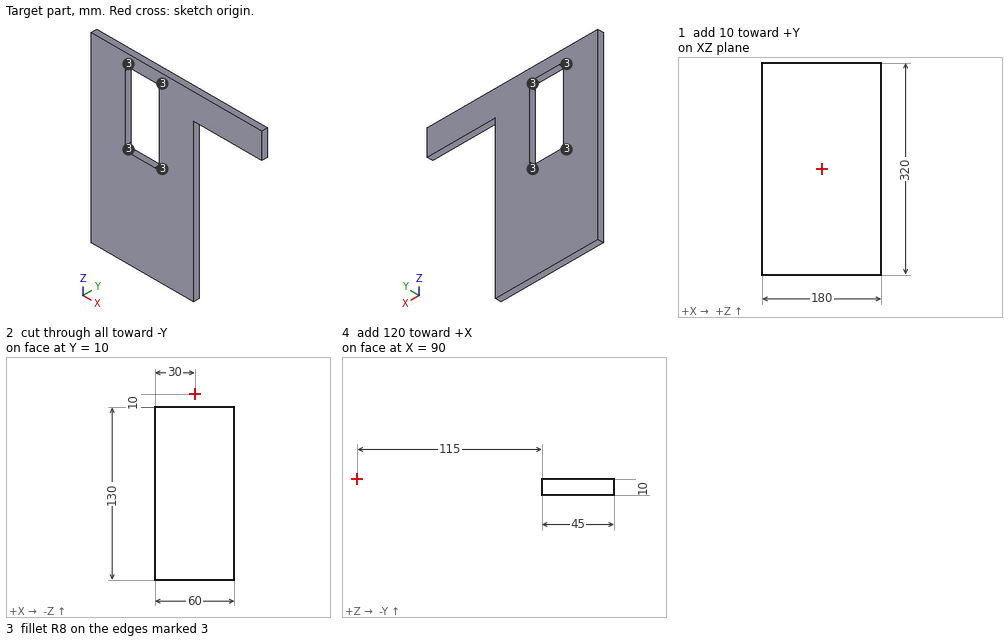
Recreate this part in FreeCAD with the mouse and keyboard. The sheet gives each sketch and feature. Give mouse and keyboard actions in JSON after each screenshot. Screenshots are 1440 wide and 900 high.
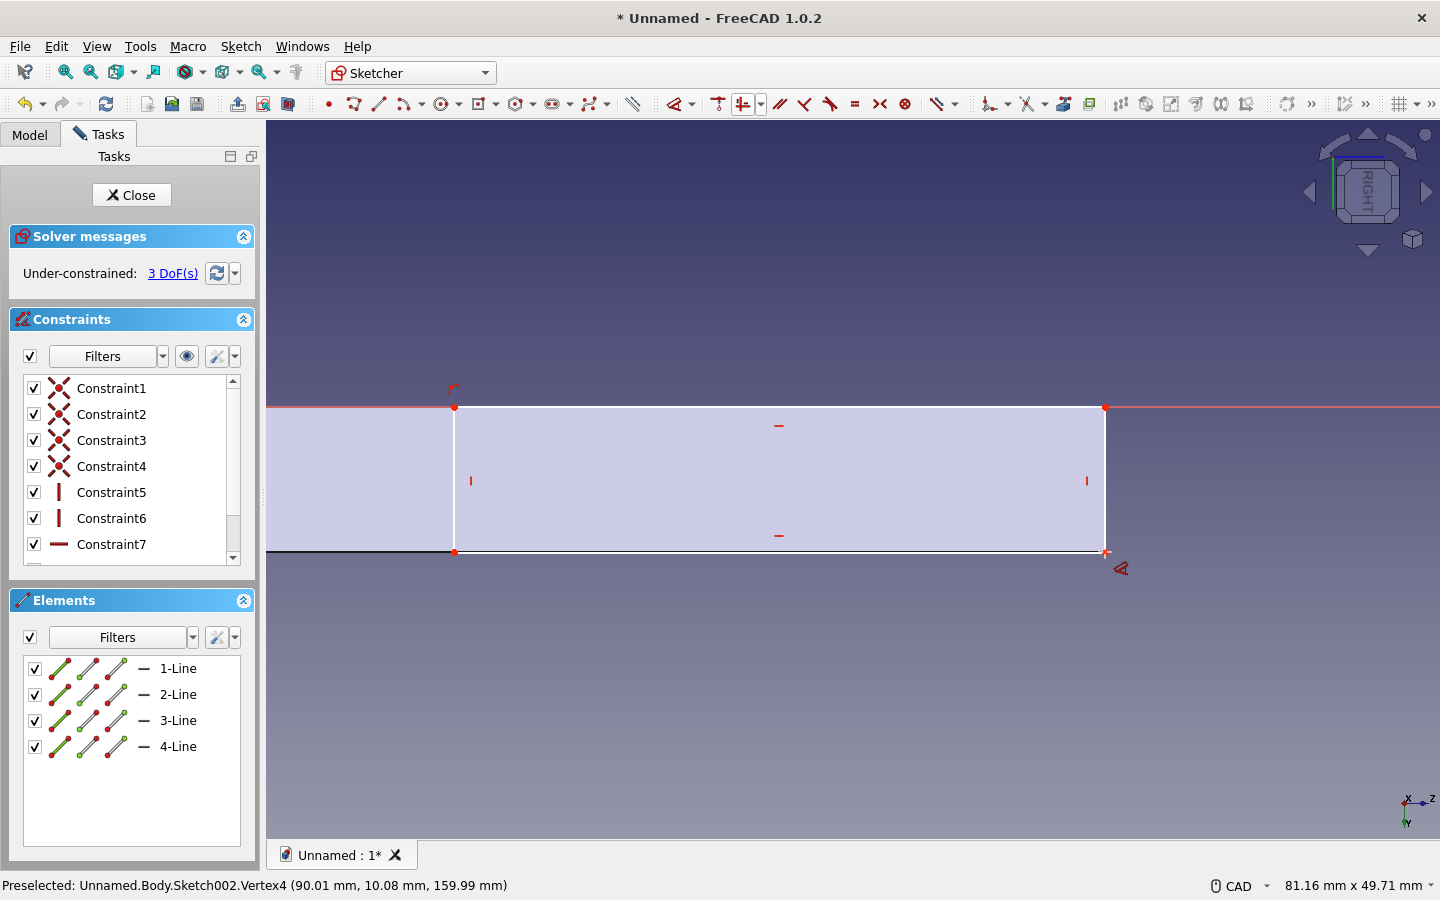
{"action": "left_click", "coordinate": [454, 451]}
{"action": "left_click", "coordinate": [420, 480]}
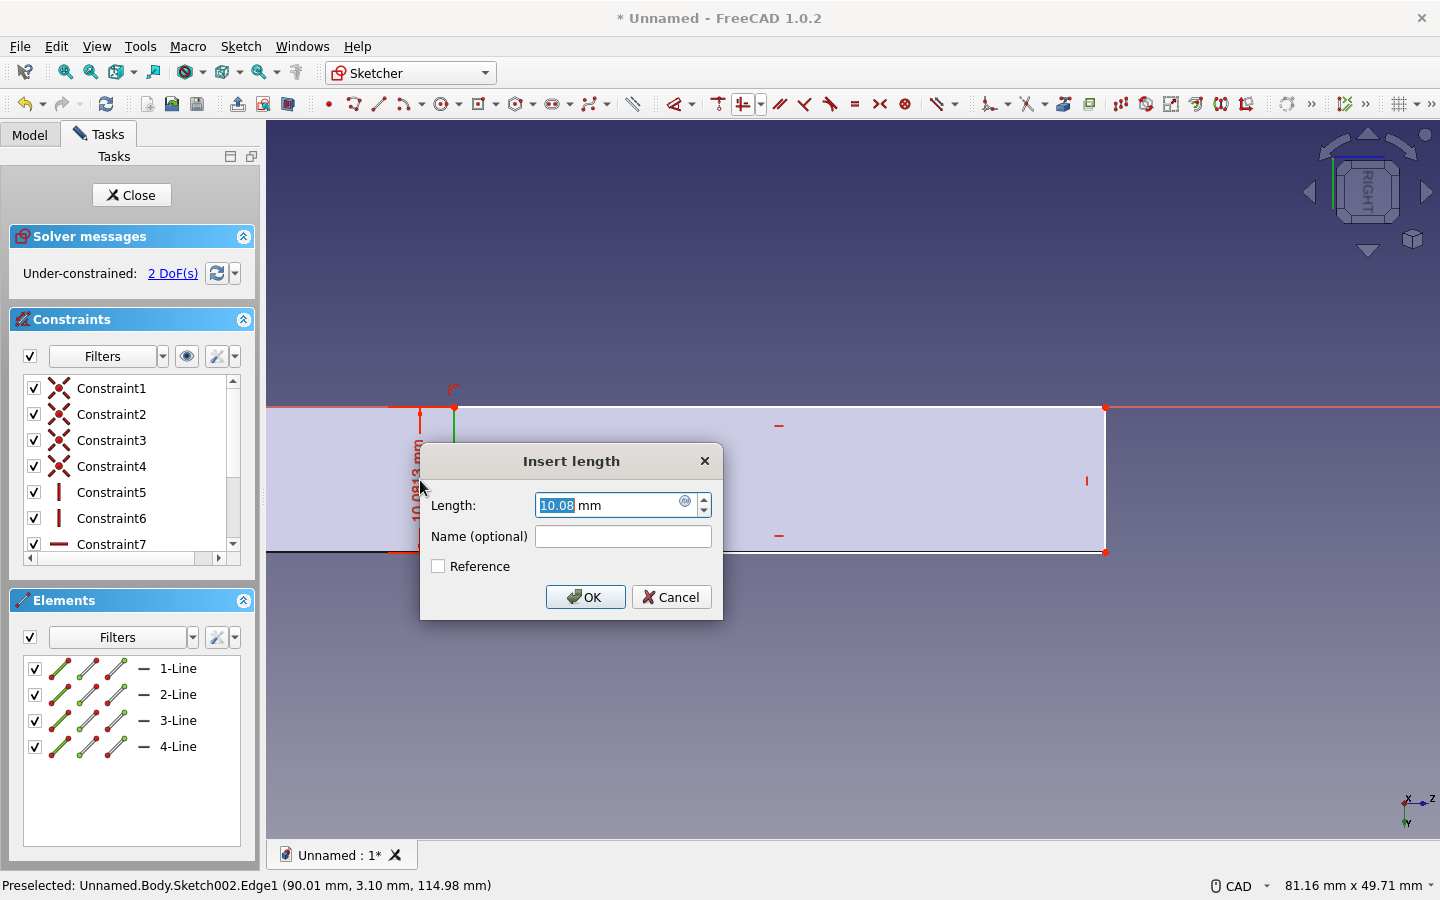
{"action": "type", "text": "10"}
{"action": "key", "text": "Return"}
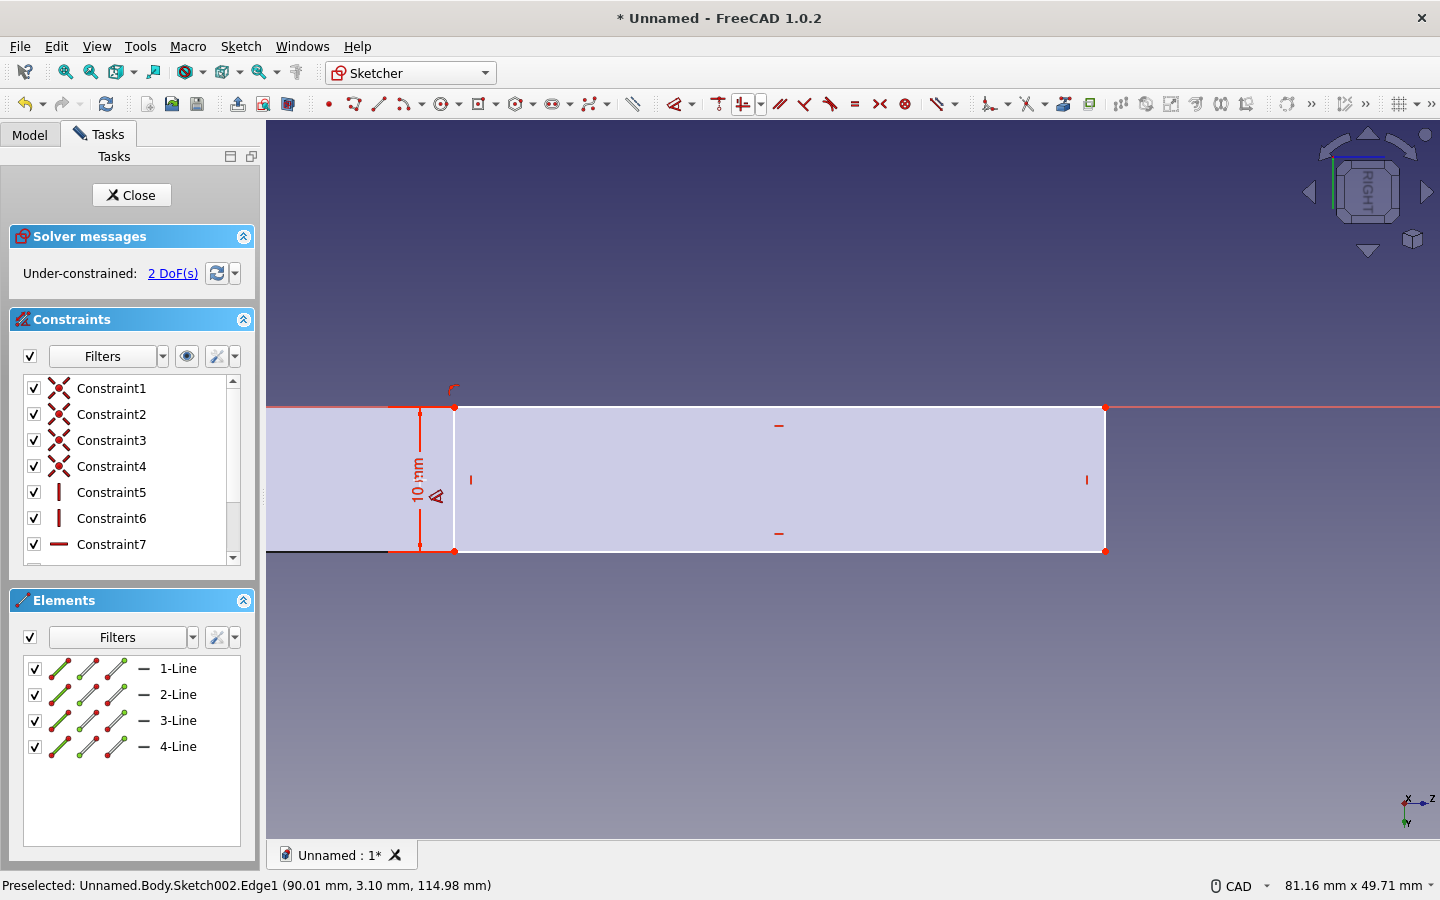
{"action": "left_click", "coordinate": [649, 552]}
{"action": "left_click", "coordinate": [779, 586]}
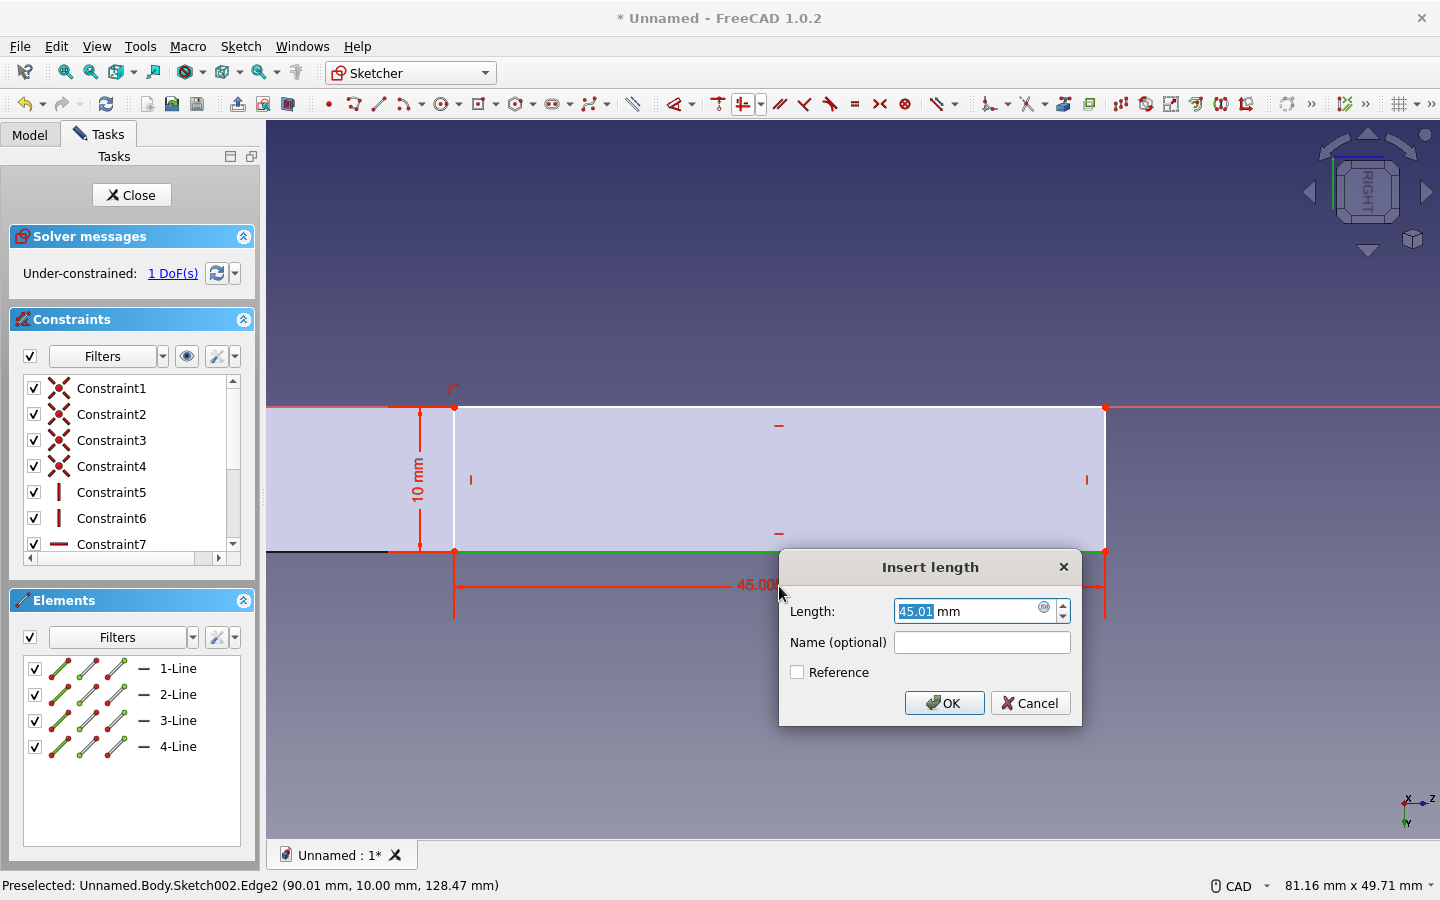
{"action": "type", "text": "45"}
{"action": "key", "text": "Return"}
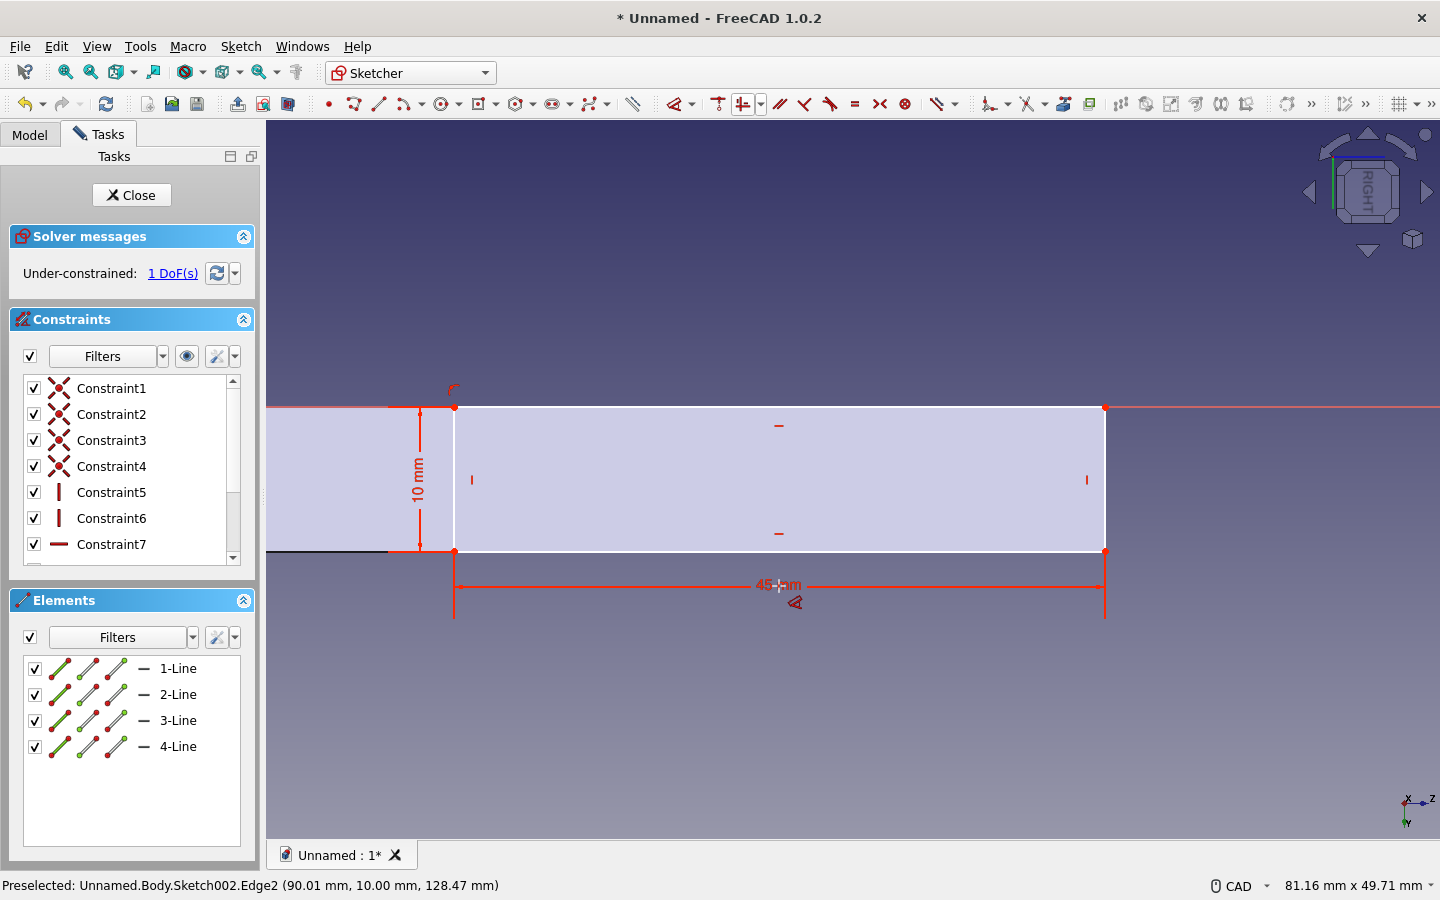
{"action": "left_click", "coordinate": [454, 407]}
{"action": "left_click", "coordinate": [374, 373]}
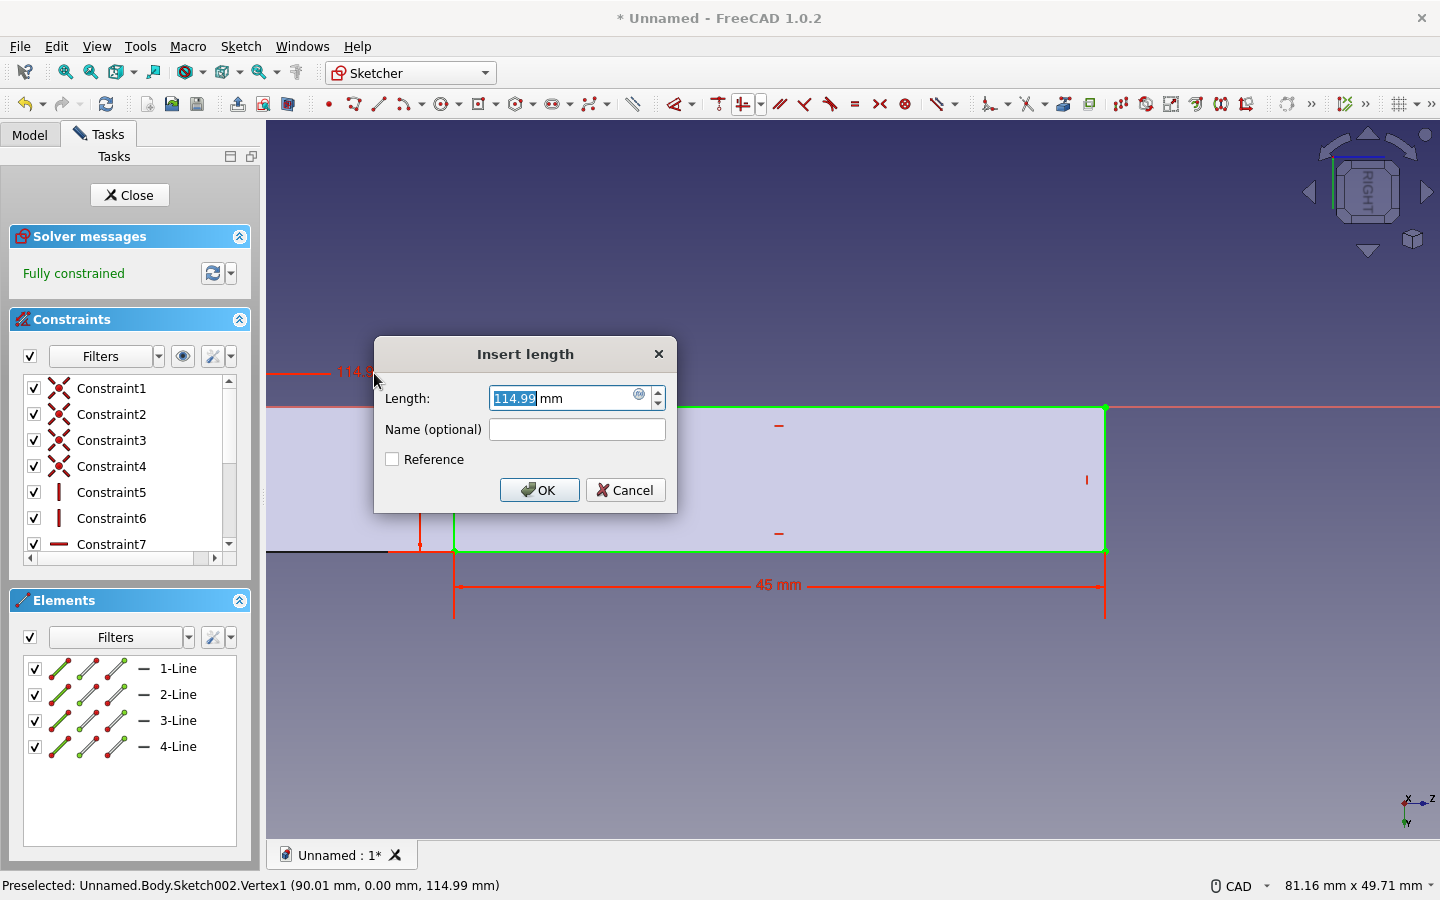
{"action": "type", "text": "115"}
{"action": "key", "text": "Return"}
{"action": "key", "text": "Escape"}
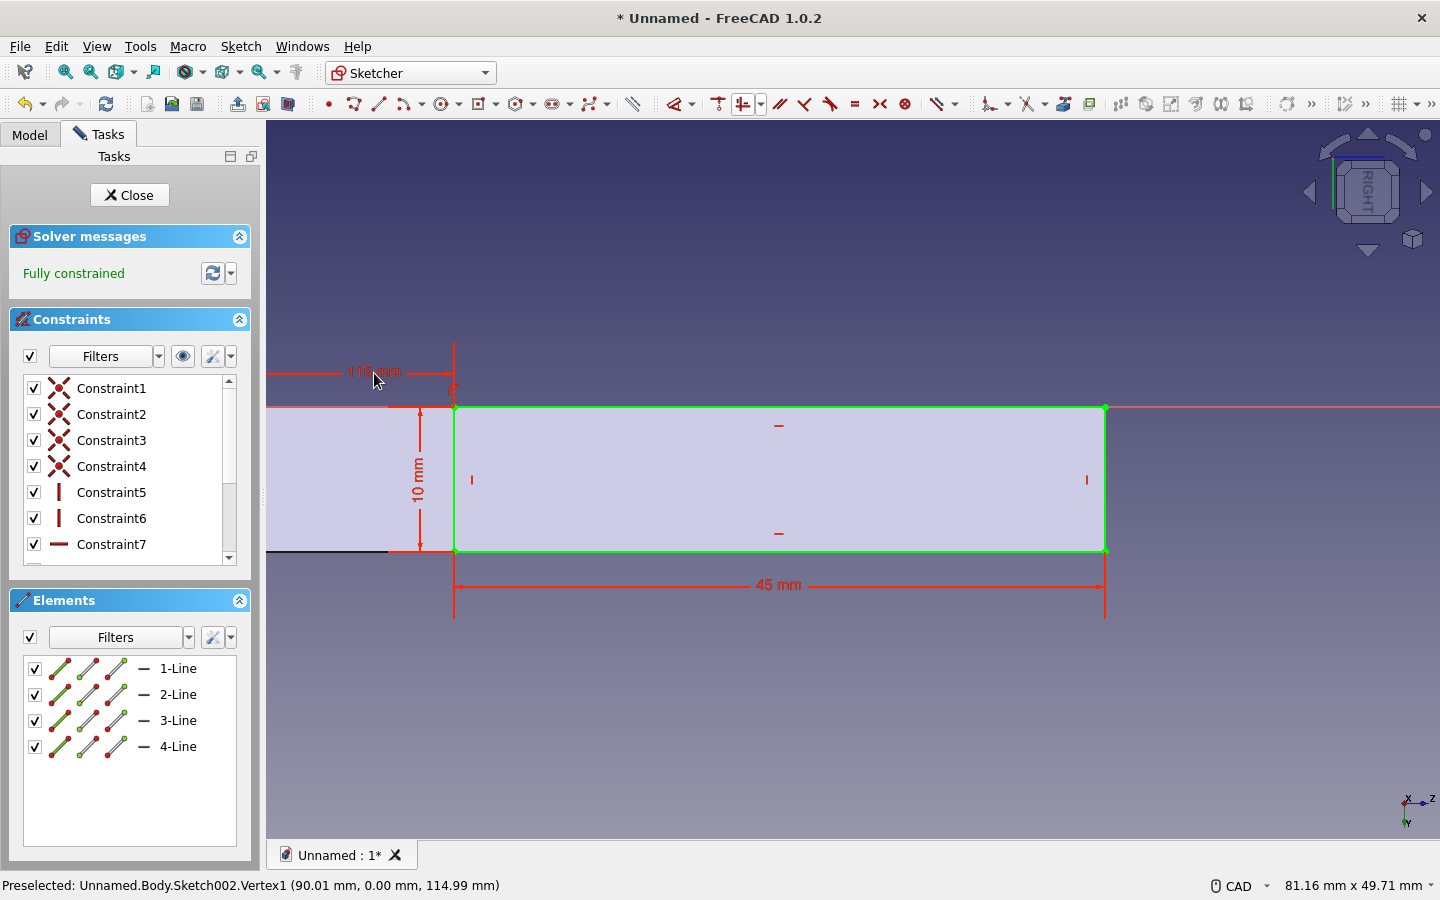
{"action": "left_click", "coordinate": [130, 195]}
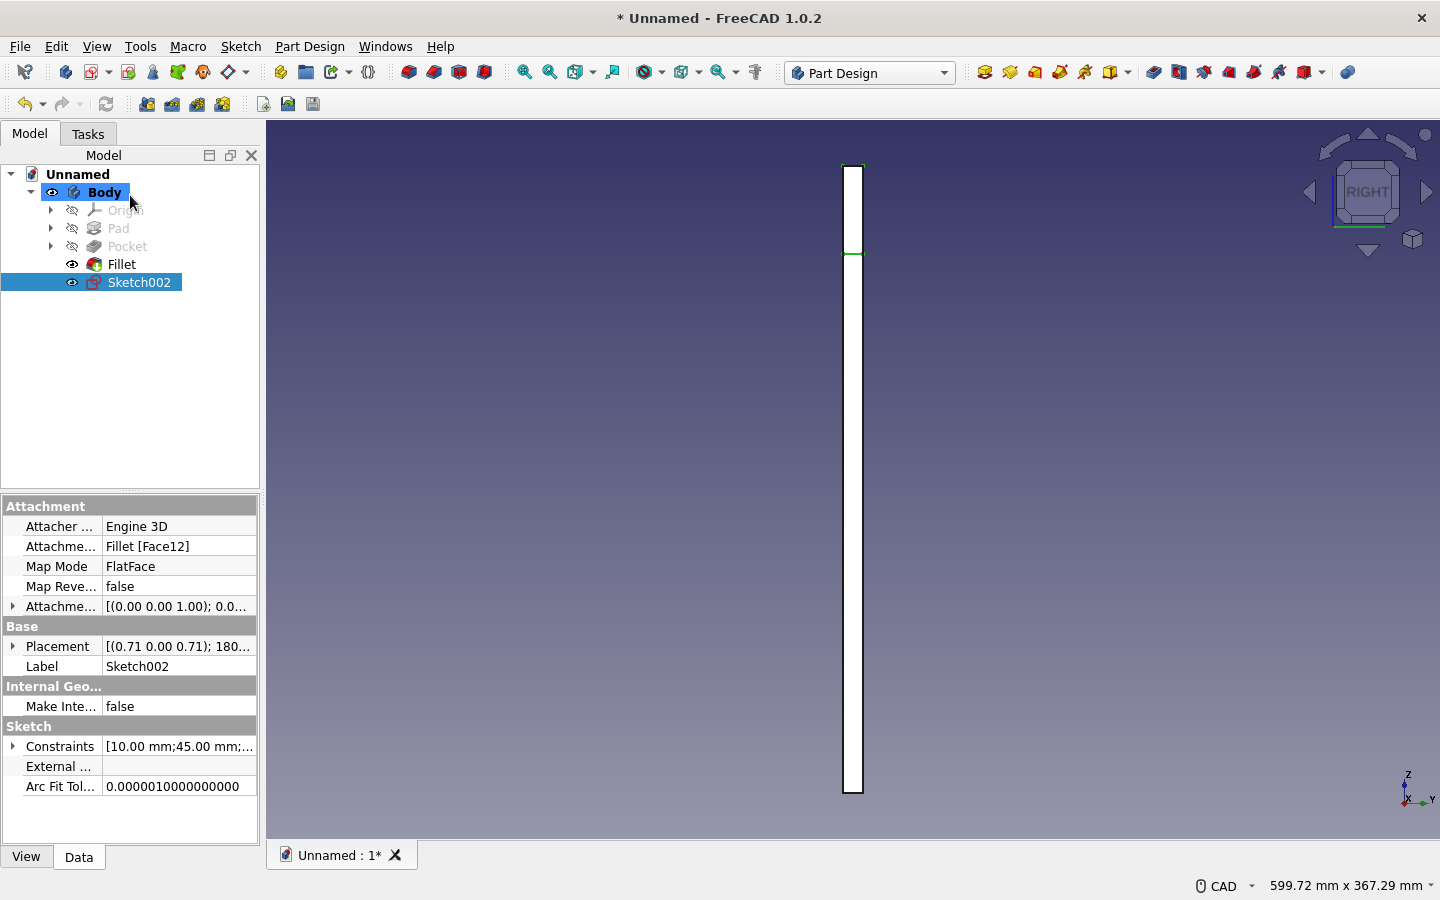
{"action": "left_click", "coordinate": [985, 72]}